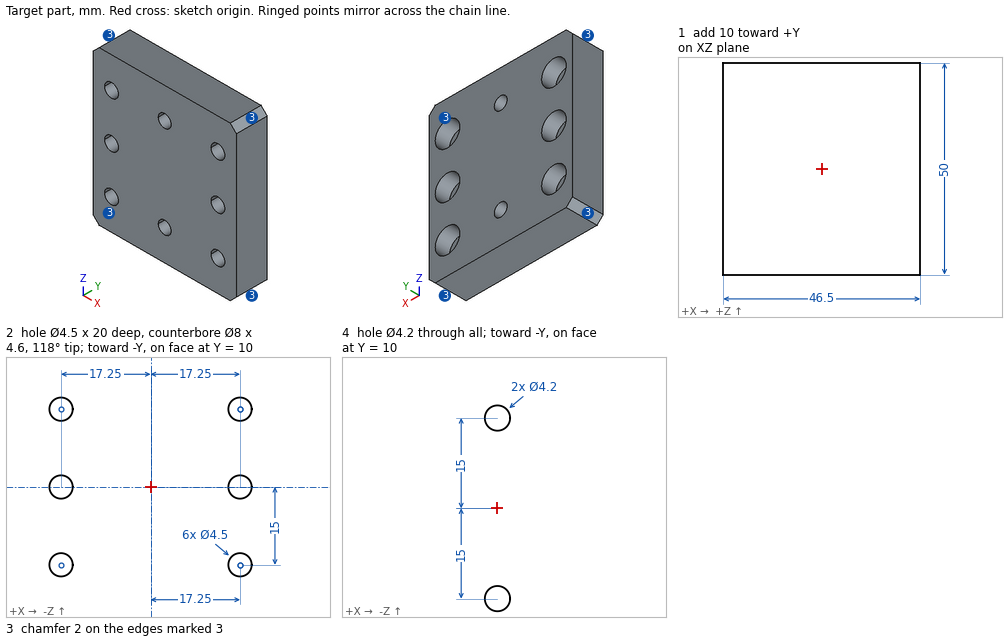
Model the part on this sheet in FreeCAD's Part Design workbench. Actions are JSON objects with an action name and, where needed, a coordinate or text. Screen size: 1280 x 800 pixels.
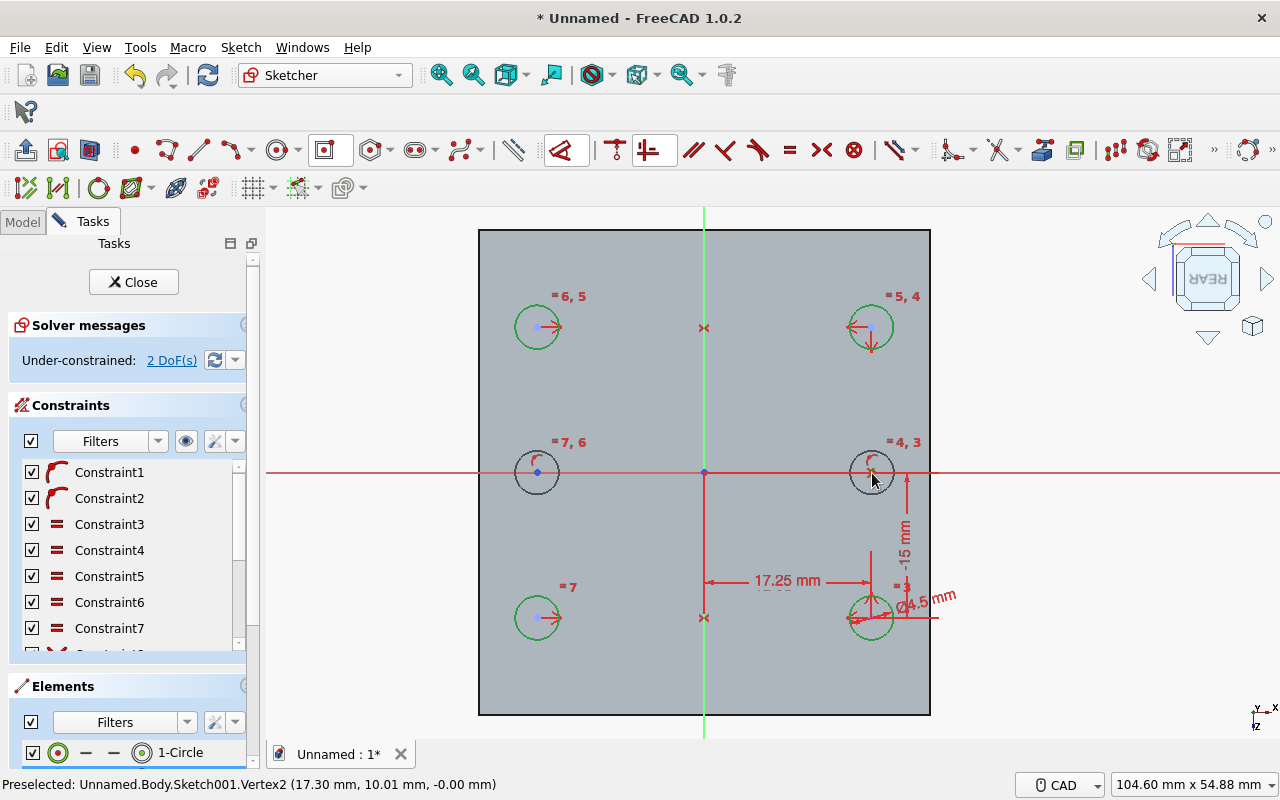
{"action": "key", "text": "l"}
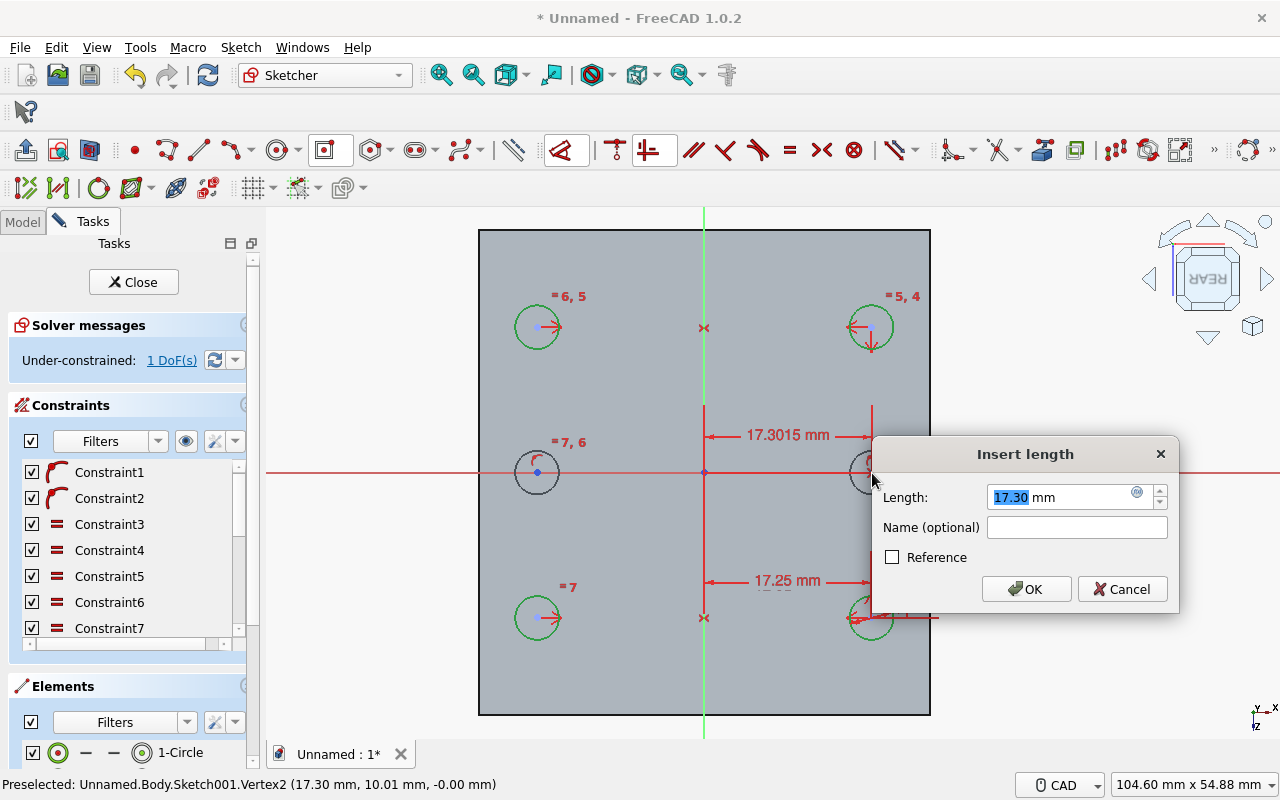
{"action": "type", "text": "17.25"}
{"action": "key", "text": "Return"}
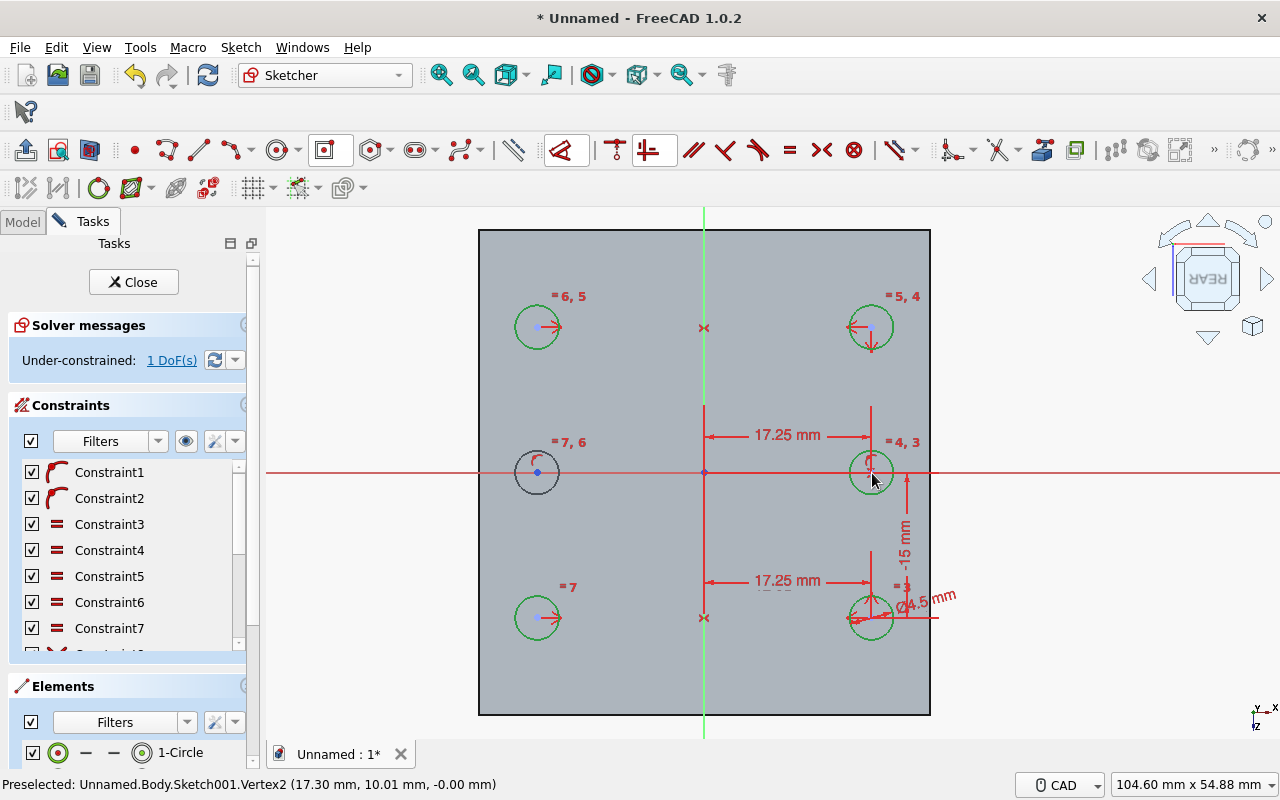
{"action": "left_click", "coordinate": [537, 473]}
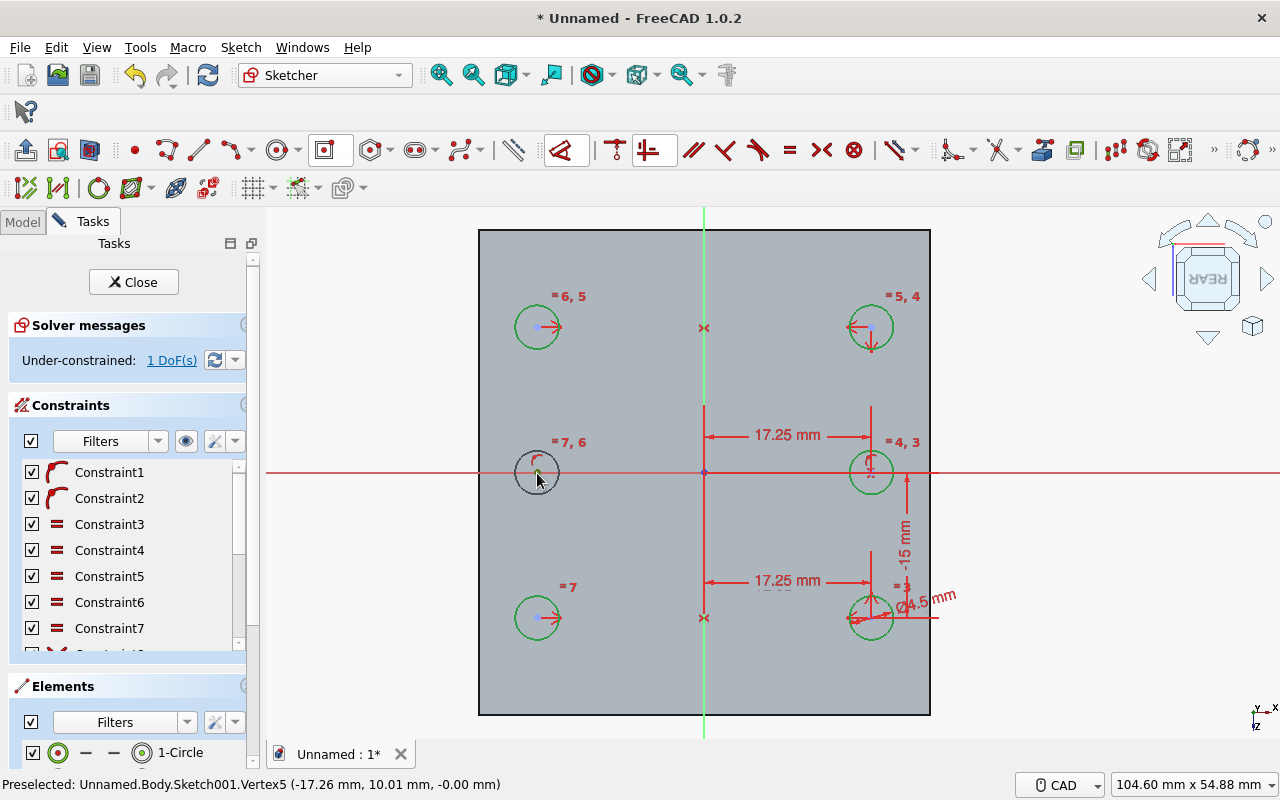
{"action": "left_click", "coordinate": [584, 150]}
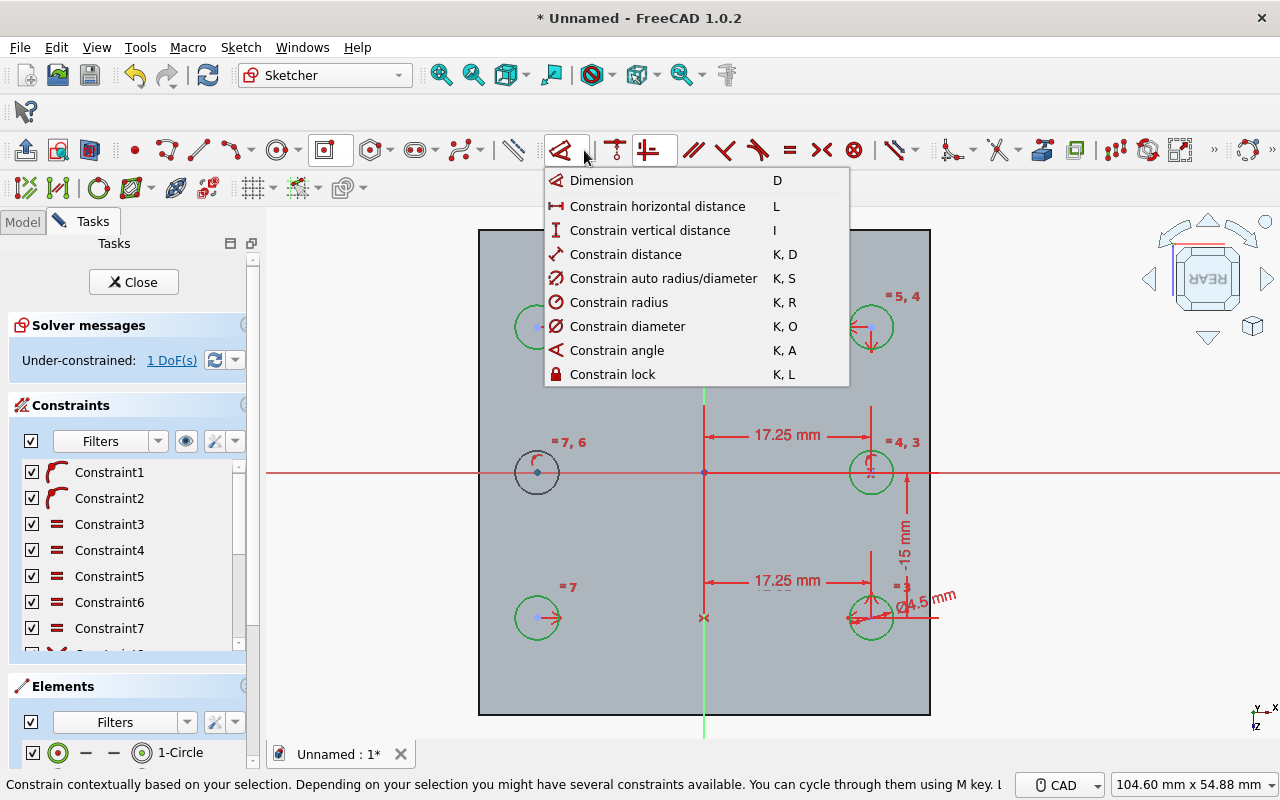
{"action": "left_click", "coordinate": [697, 206]}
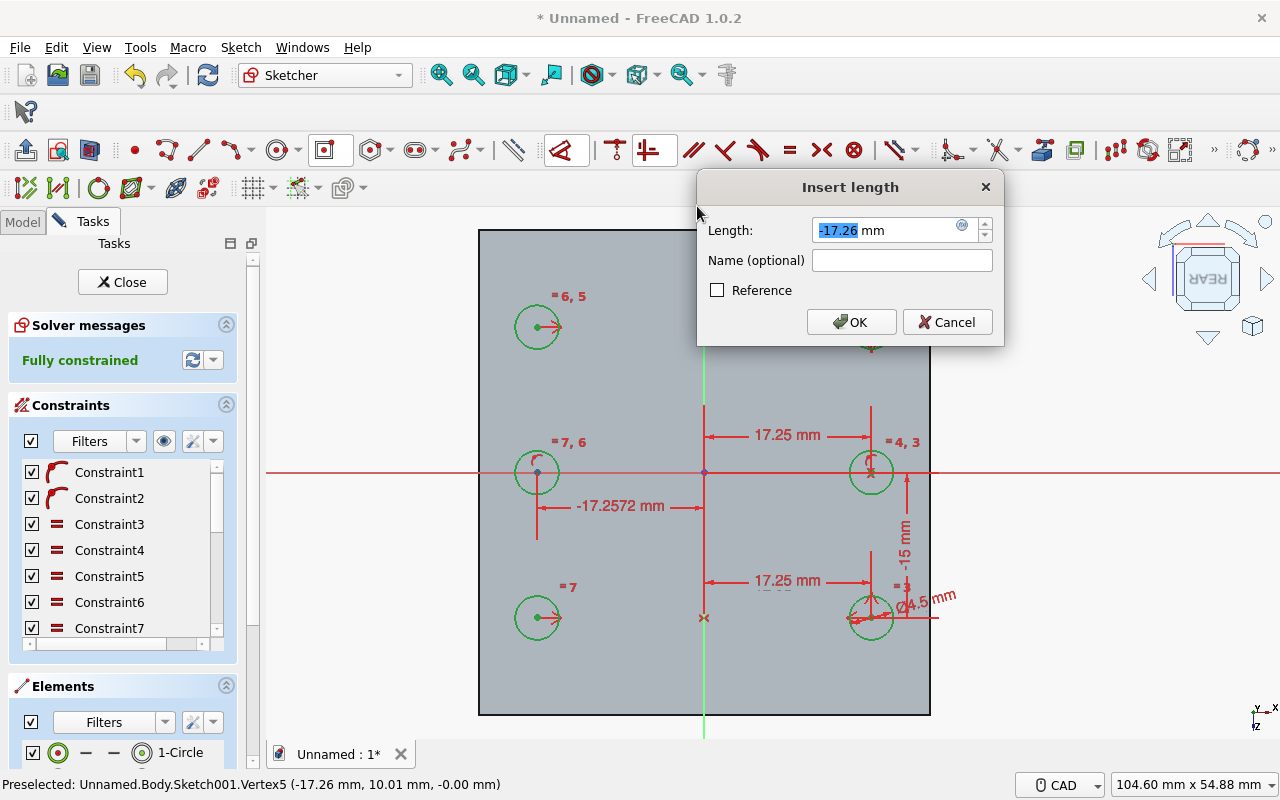
{"action": "type", "text": "-17.25"}
{"action": "key", "text": "Return"}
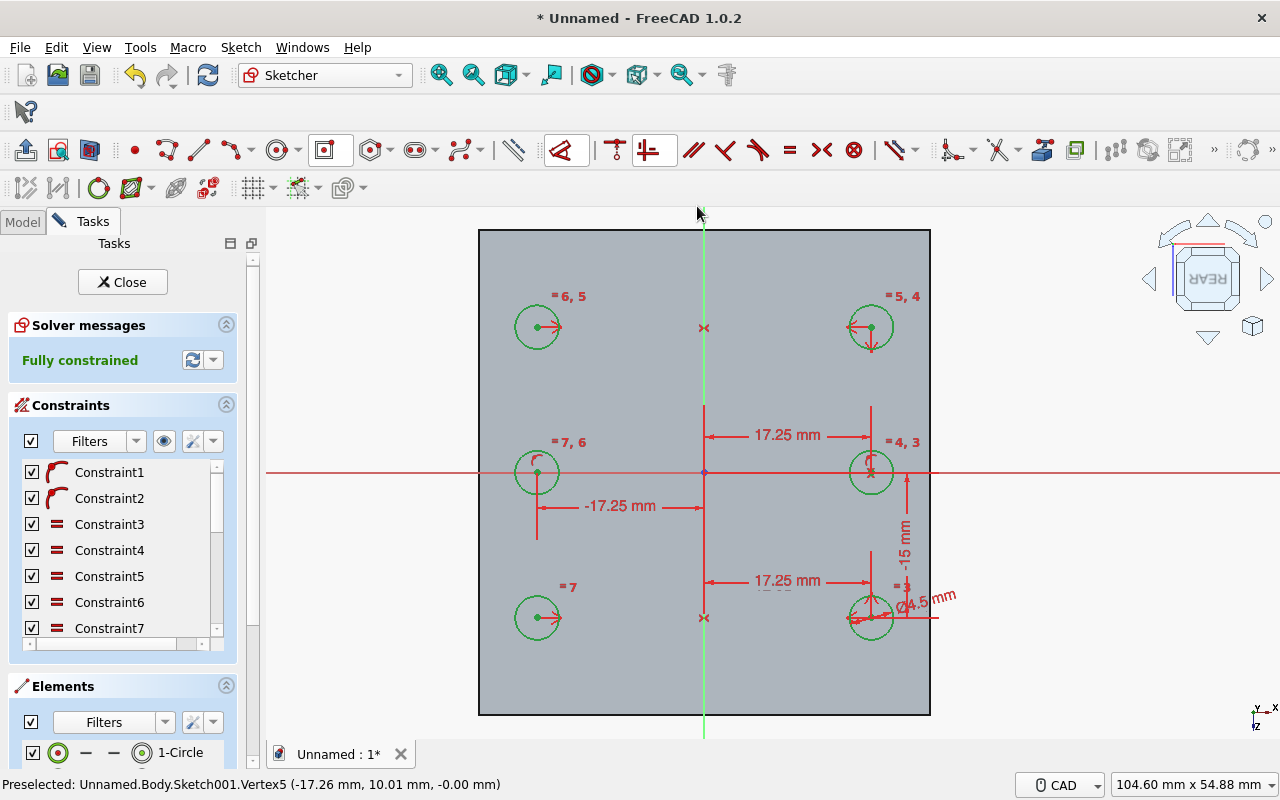
{"action": "left_click", "coordinate": [123, 282]}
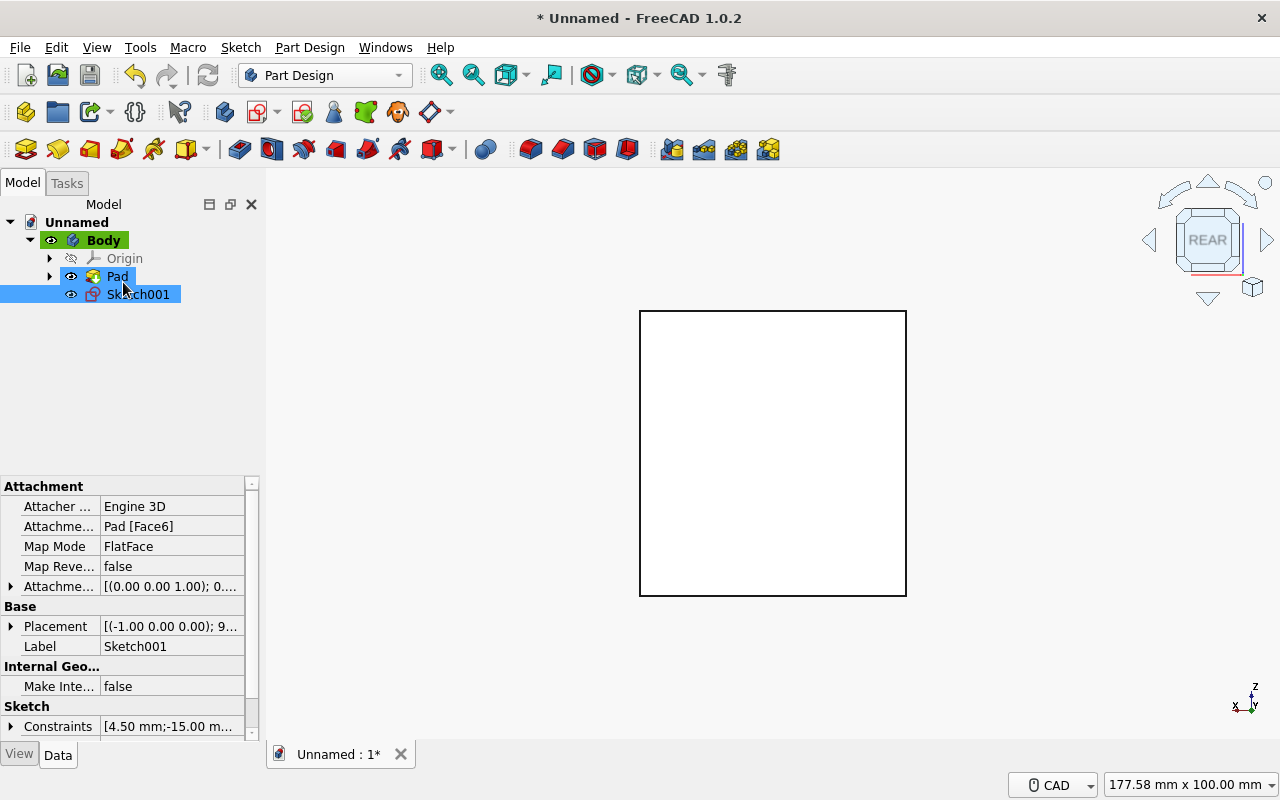
{"action": "left_click", "coordinate": [272, 150]}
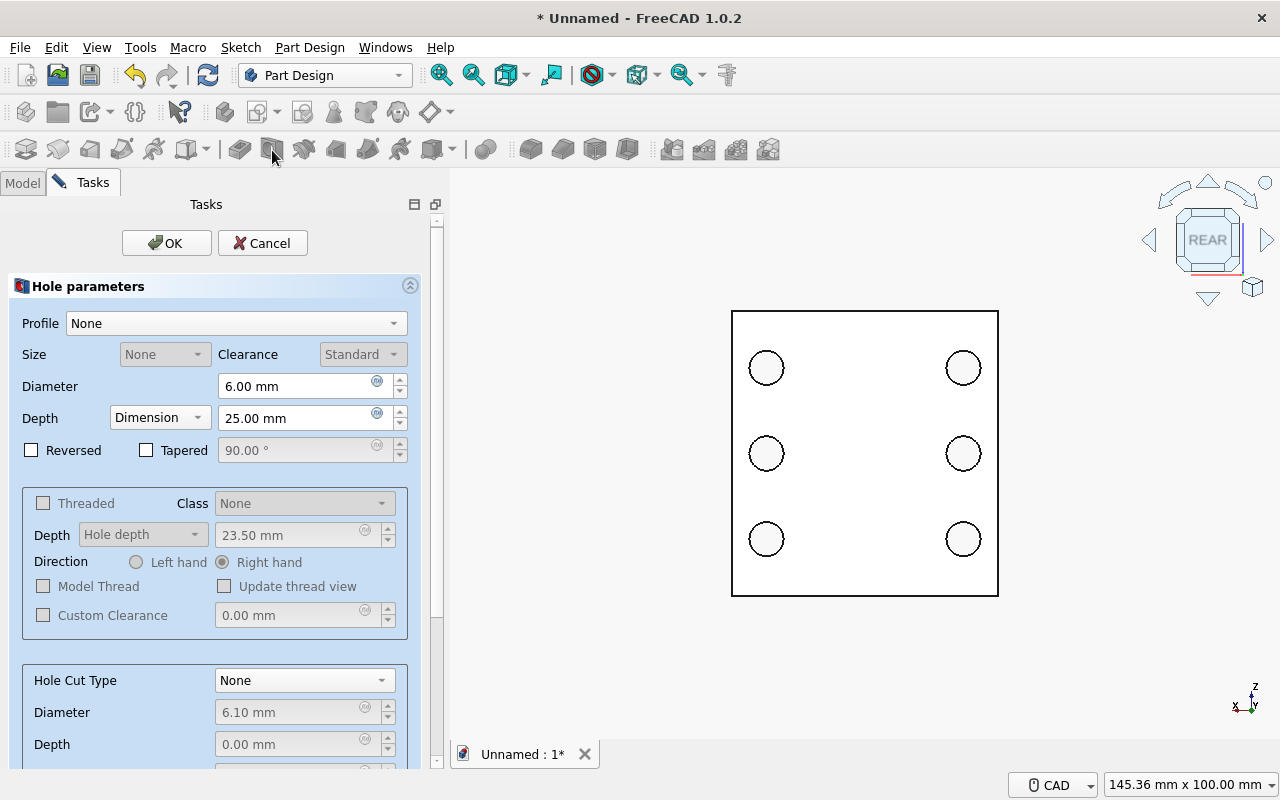
{"action": "triple_click", "coordinate": [305, 386]}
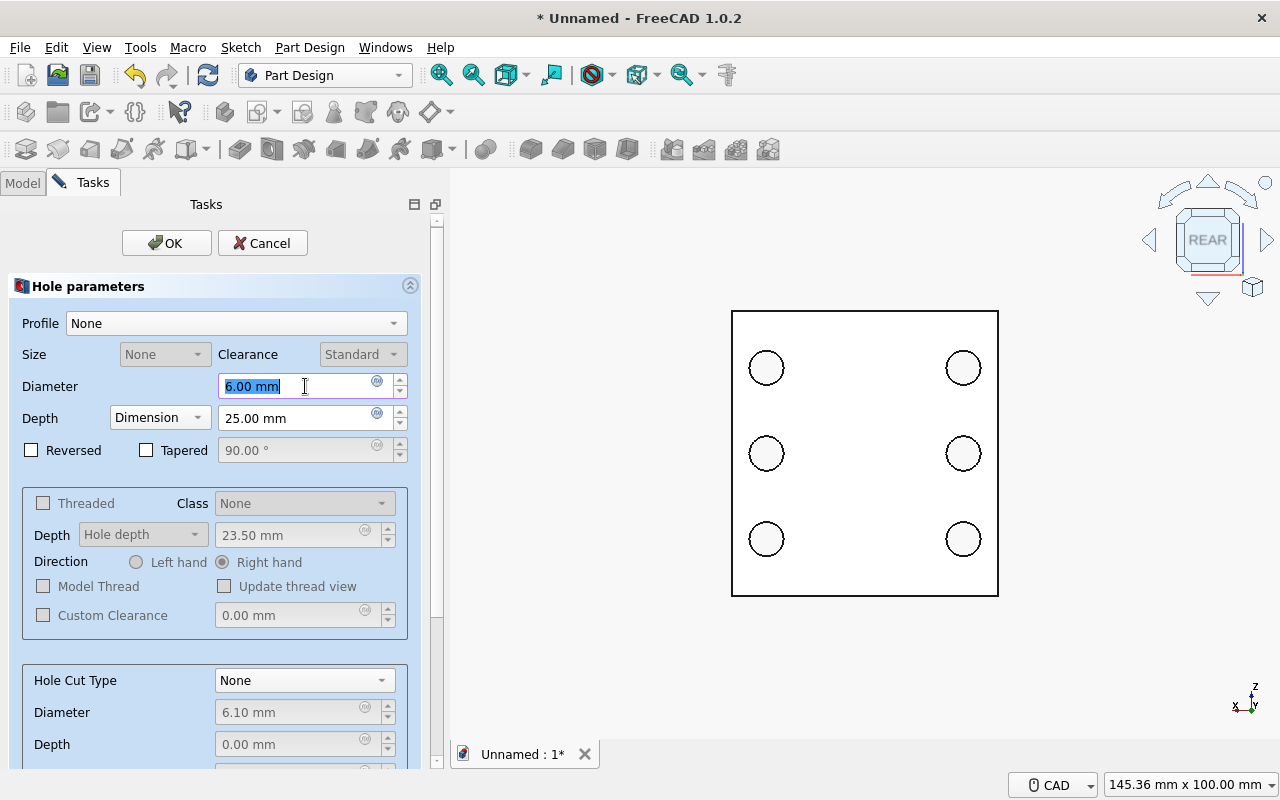
{"action": "type", "text": "4.5"}
{"action": "key", "text": "Tab"}